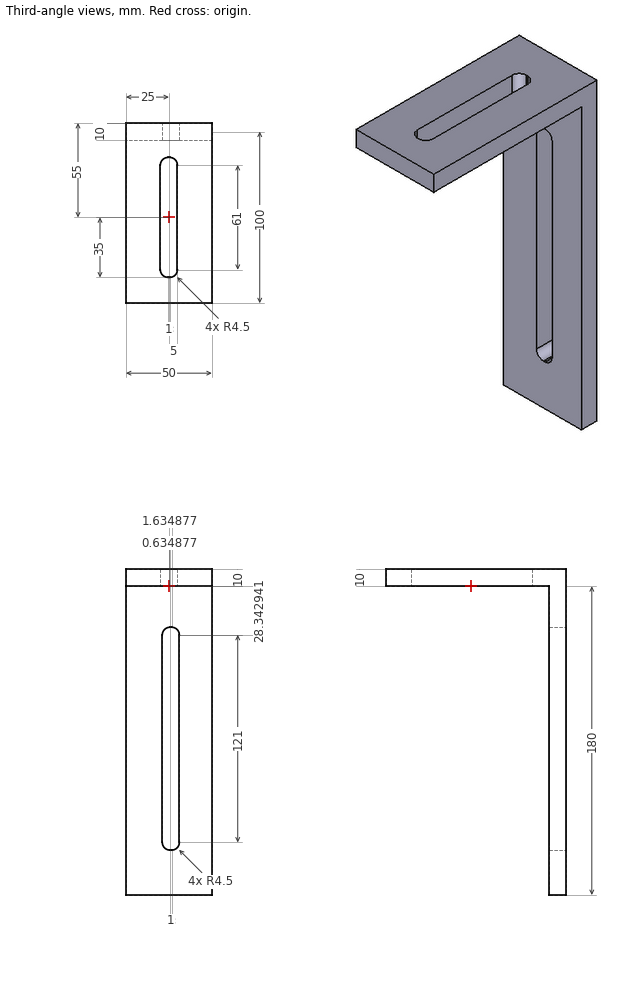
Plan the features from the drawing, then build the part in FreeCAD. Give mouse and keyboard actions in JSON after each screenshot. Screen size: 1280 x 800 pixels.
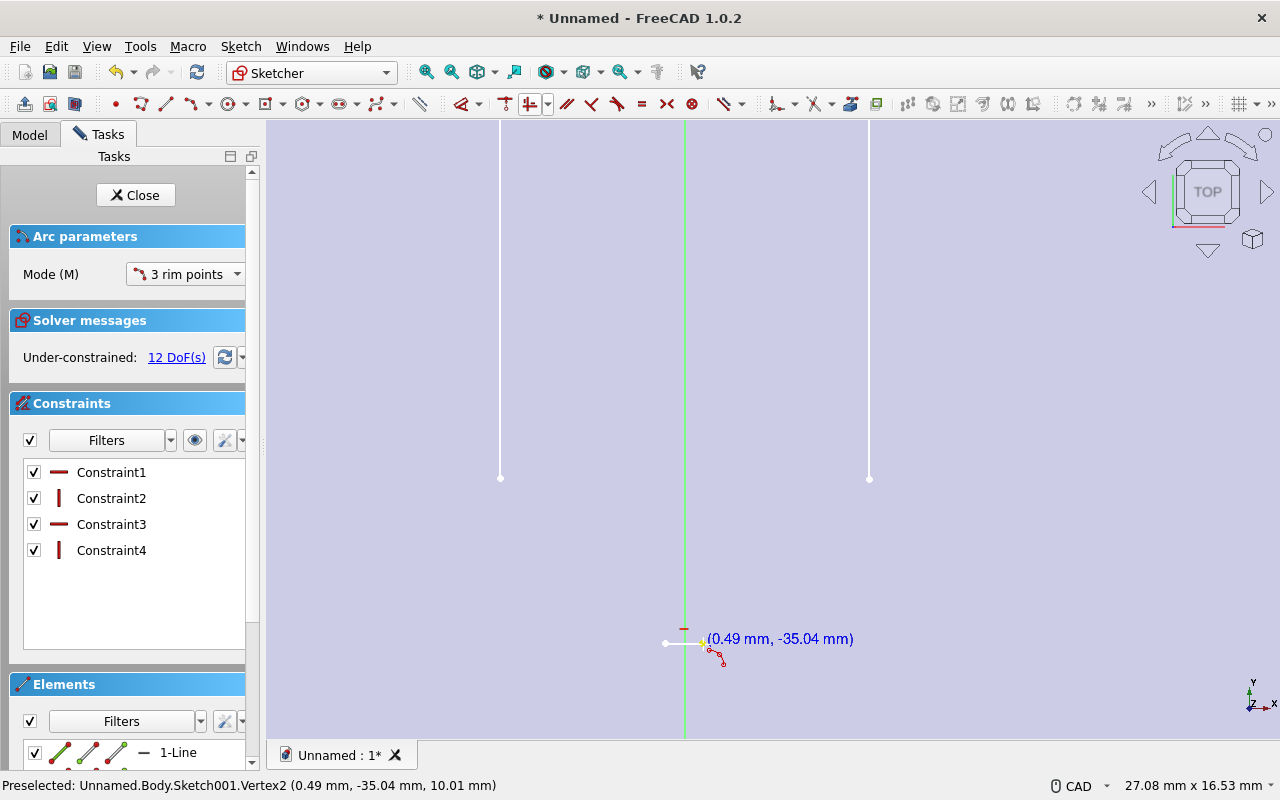
{"action": "scroll", "coordinate": [708, 647], "scroll_direction": "down", "scroll_amount": 9}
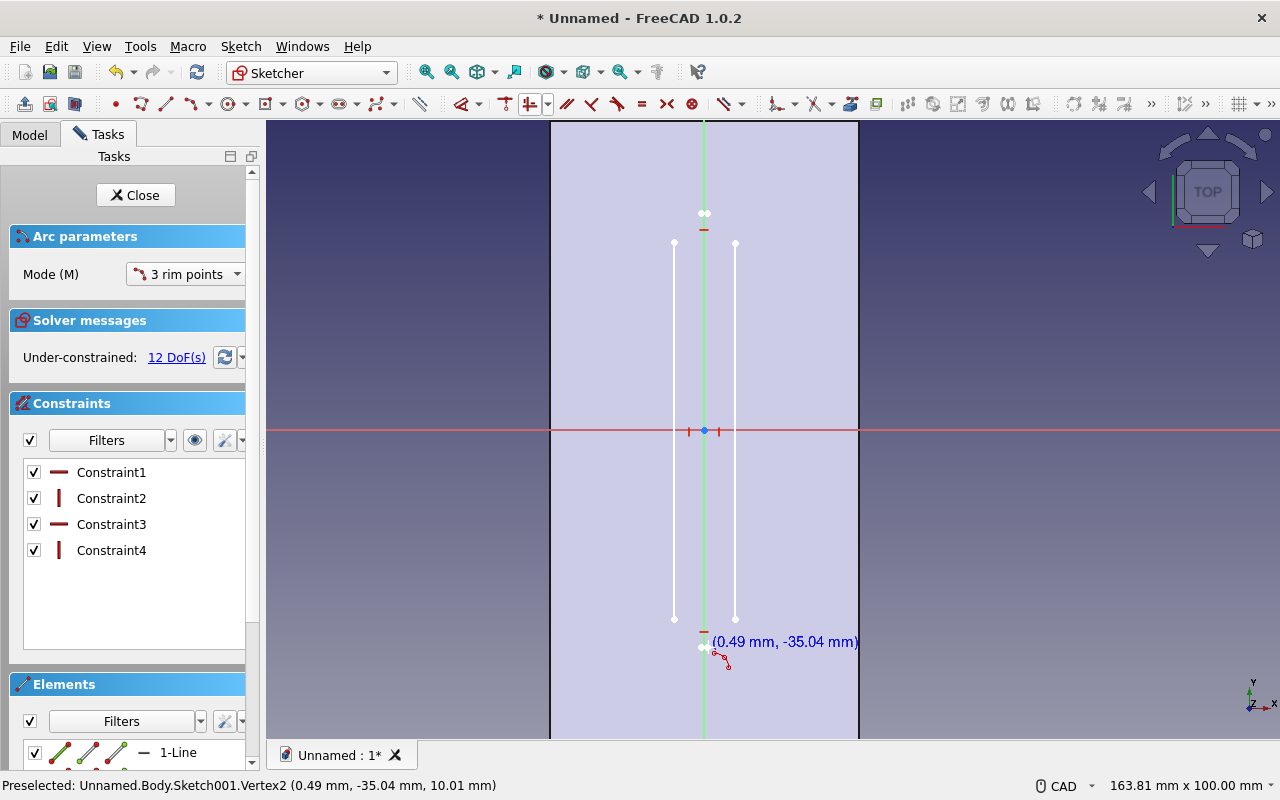
{"action": "left_click", "coordinate": [735, 620]}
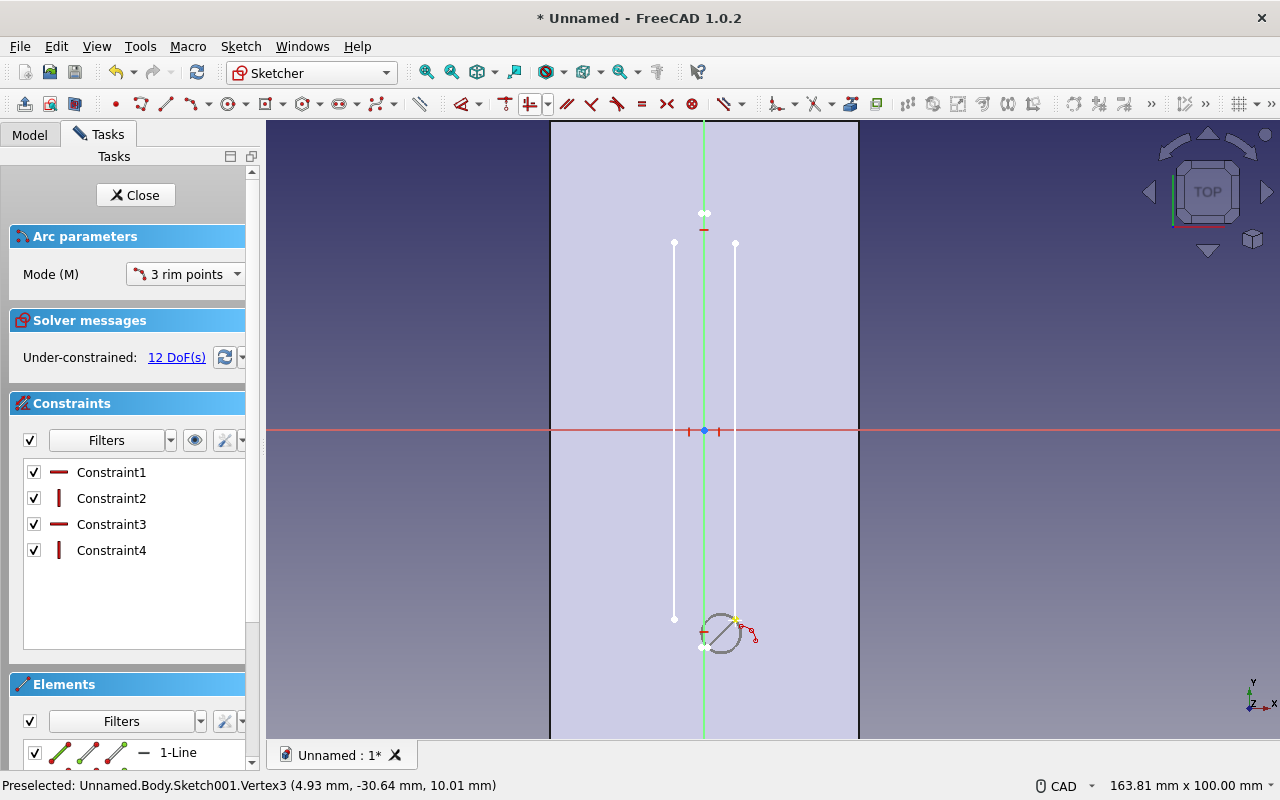
{"action": "scroll", "coordinate": [727, 639], "scroll_direction": "up", "scroll_amount": 4}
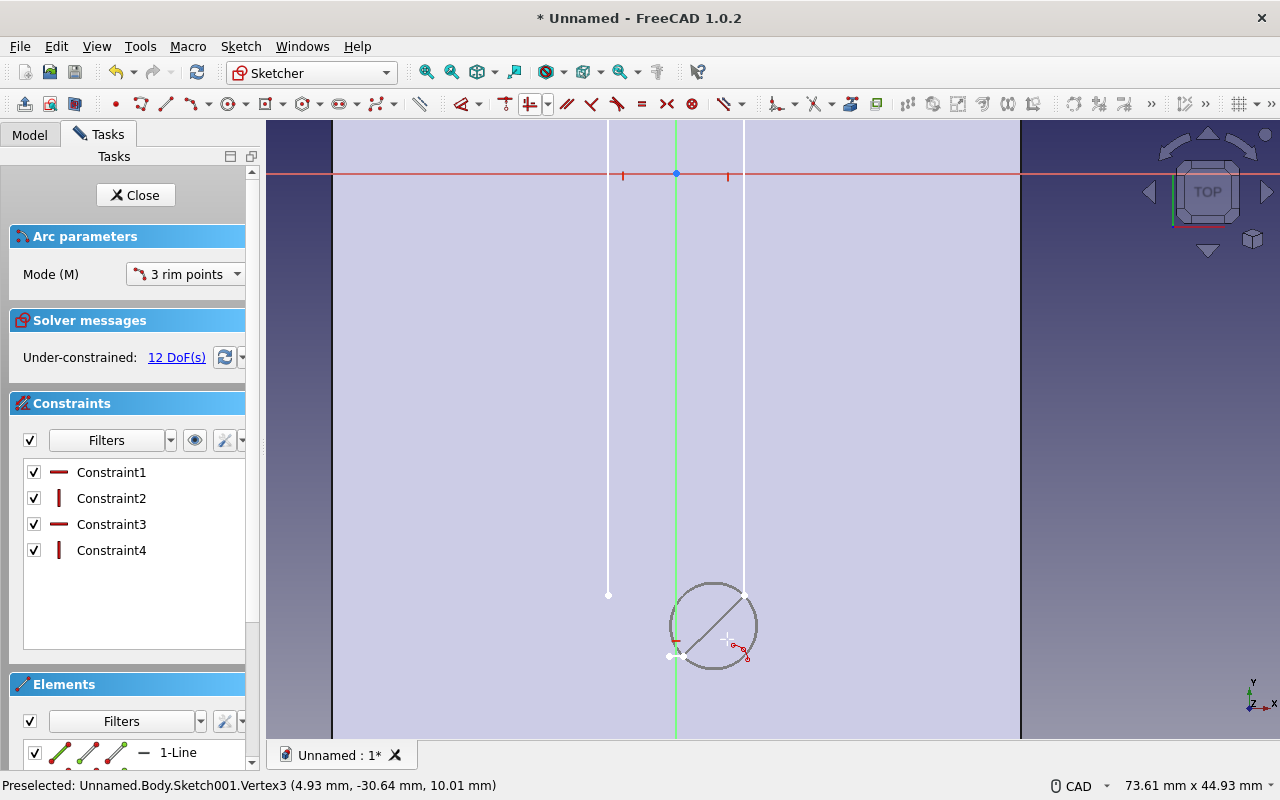
{"action": "left_click", "coordinate": [727, 638]}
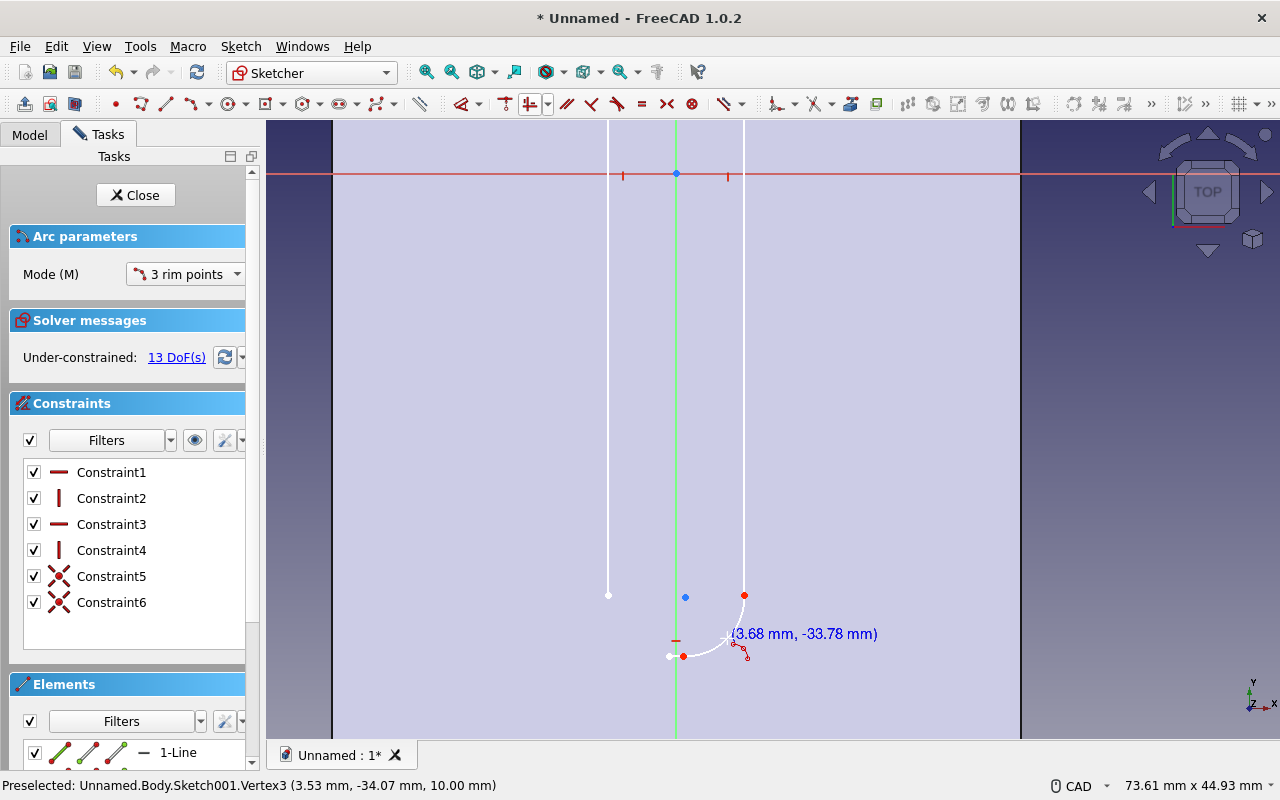
{"action": "scroll", "coordinate": [727, 638], "scroll_direction": "down", "scroll_amount": 4}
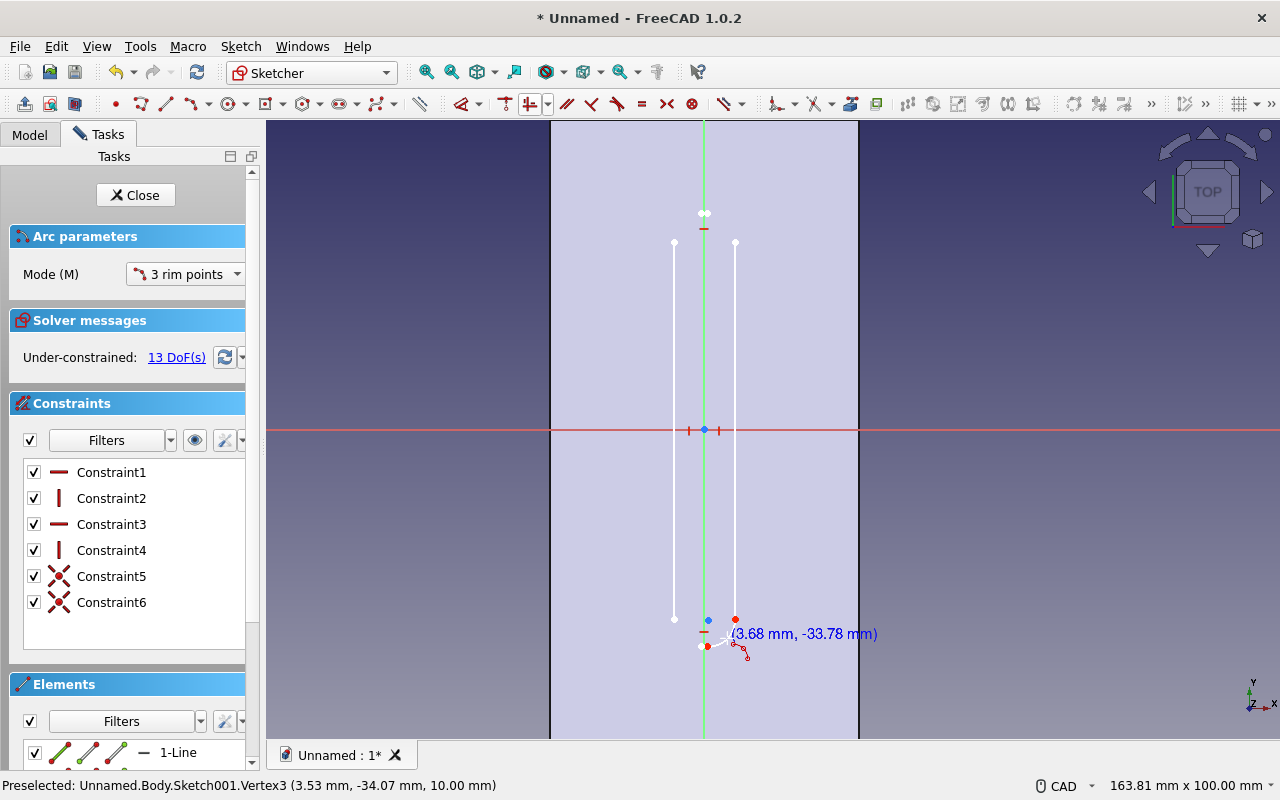
{"action": "left_click", "coordinate": [735, 242]}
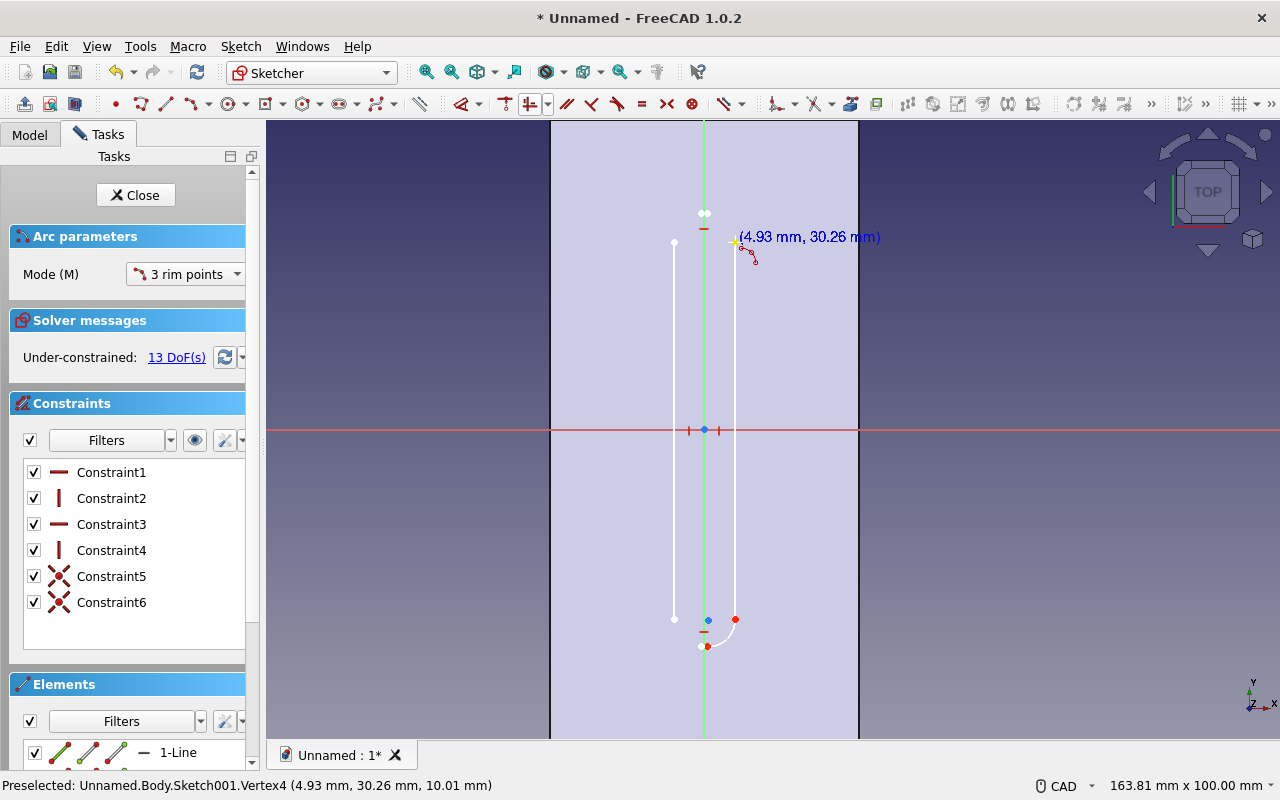
{"action": "scroll", "coordinate": [708, 213], "scroll_direction": "up", "scroll_amount": 9}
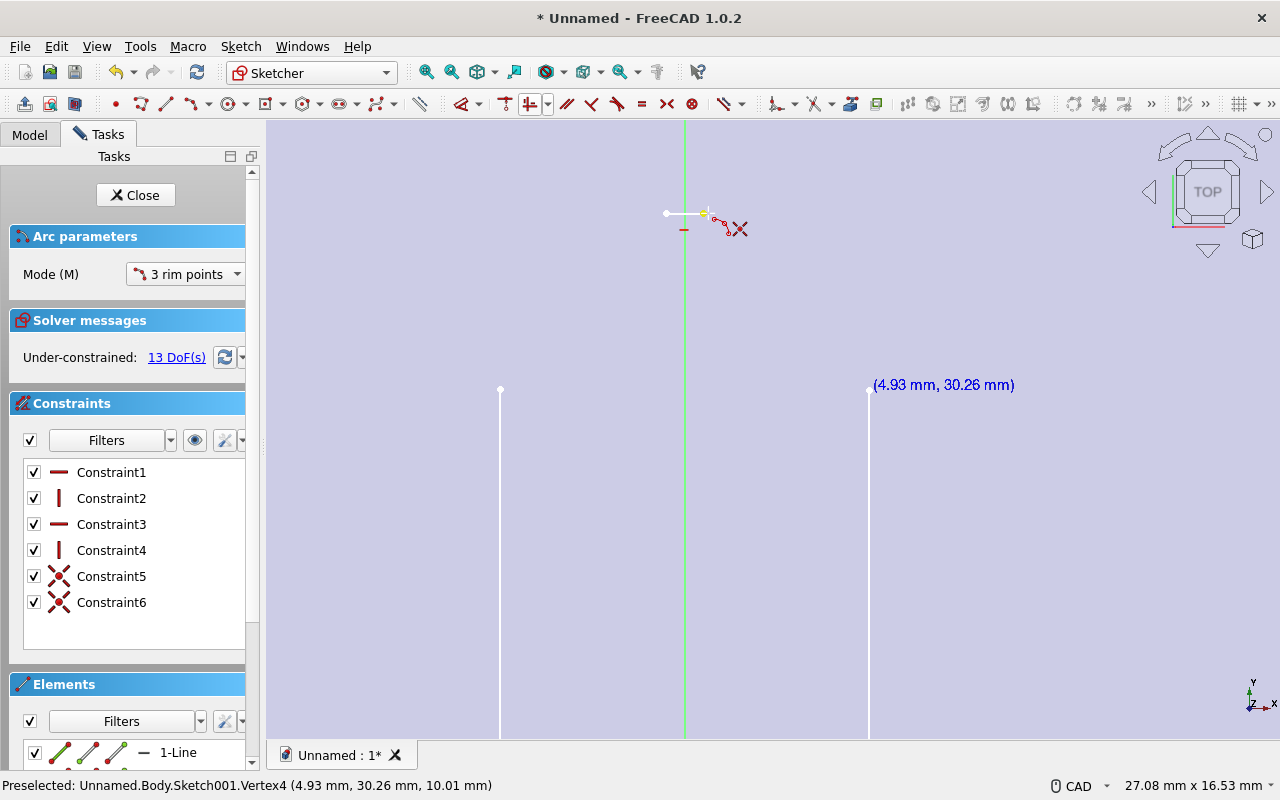
{"action": "left_click", "coordinate": [703, 214]}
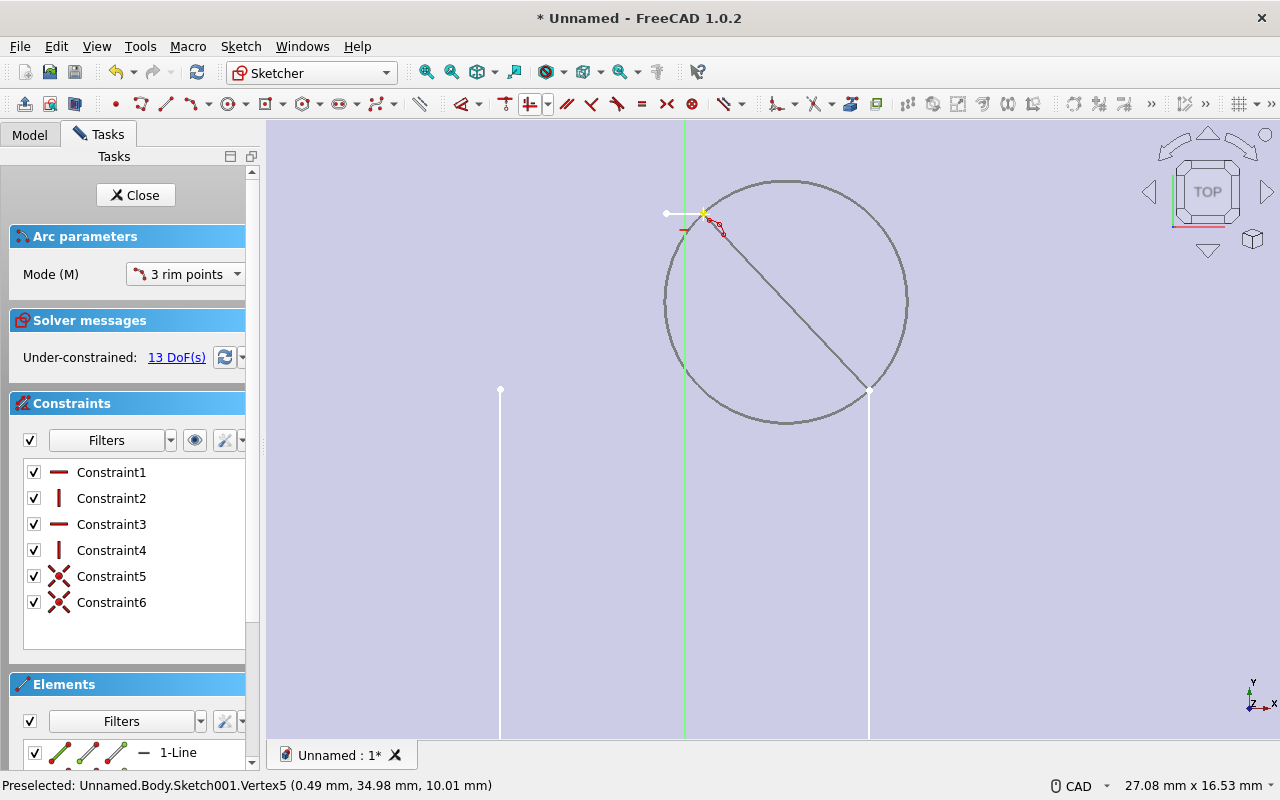
{"action": "scroll", "coordinate": [708, 213], "scroll_direction": "down", "scroll_amount": 9}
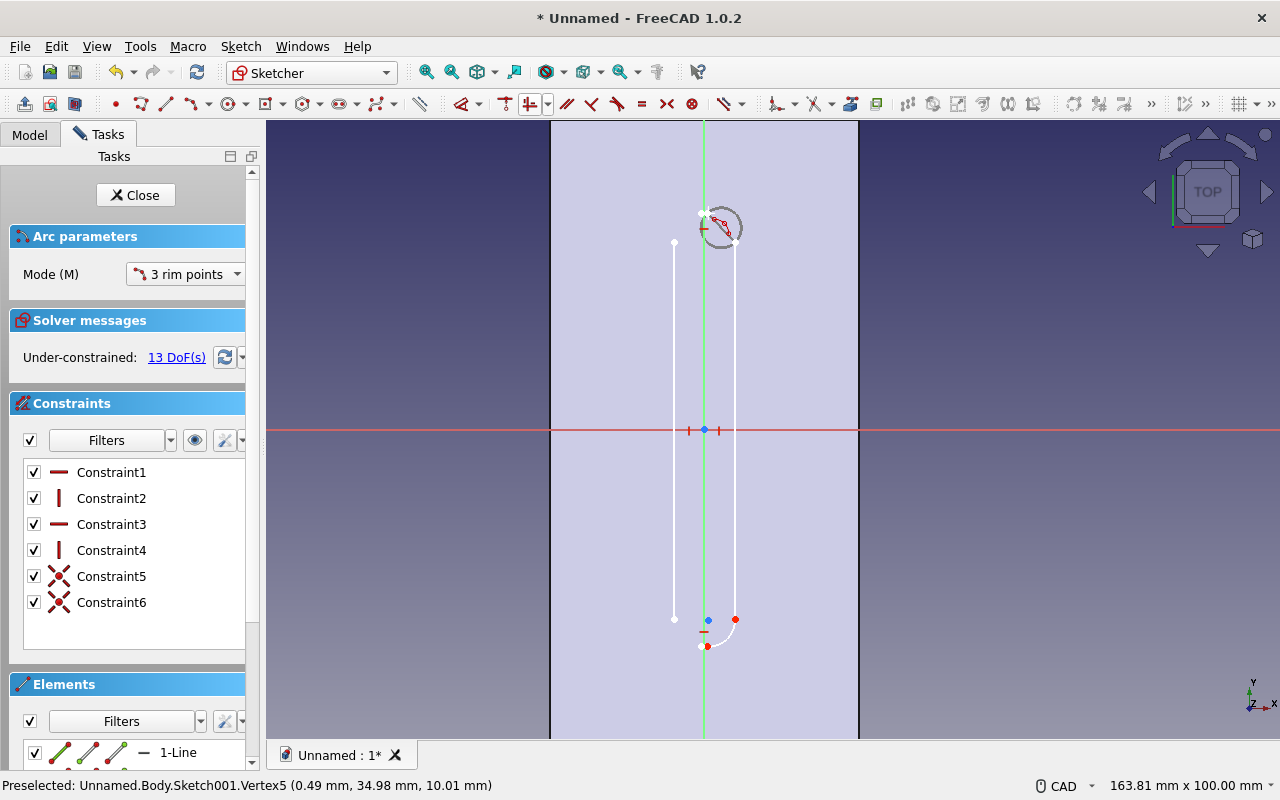
{"action": "scroll", "coordinate": [727, 221], "scroll_direction": "up", "scroll_amount": 4}